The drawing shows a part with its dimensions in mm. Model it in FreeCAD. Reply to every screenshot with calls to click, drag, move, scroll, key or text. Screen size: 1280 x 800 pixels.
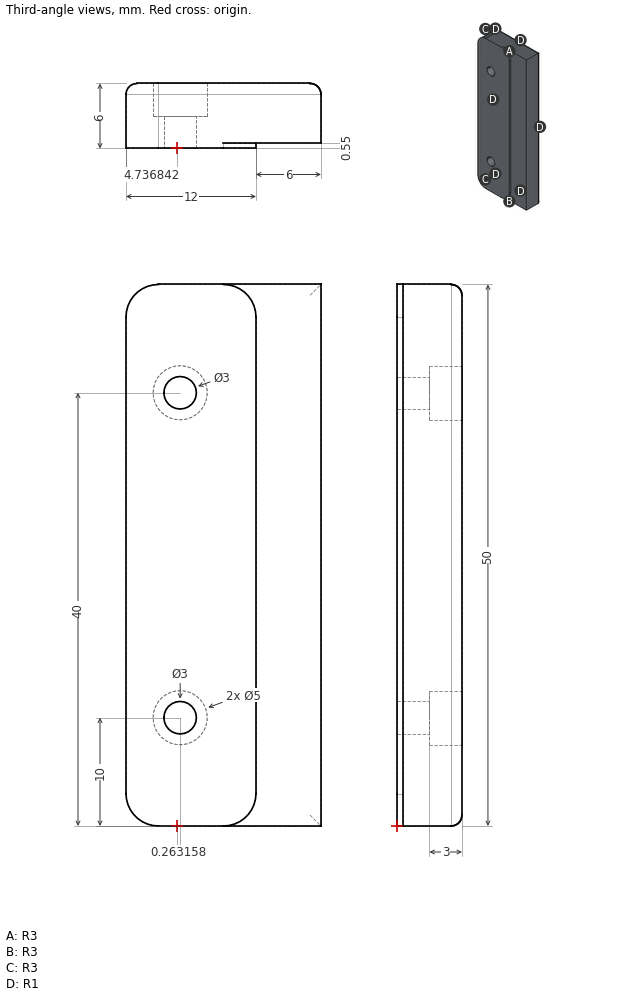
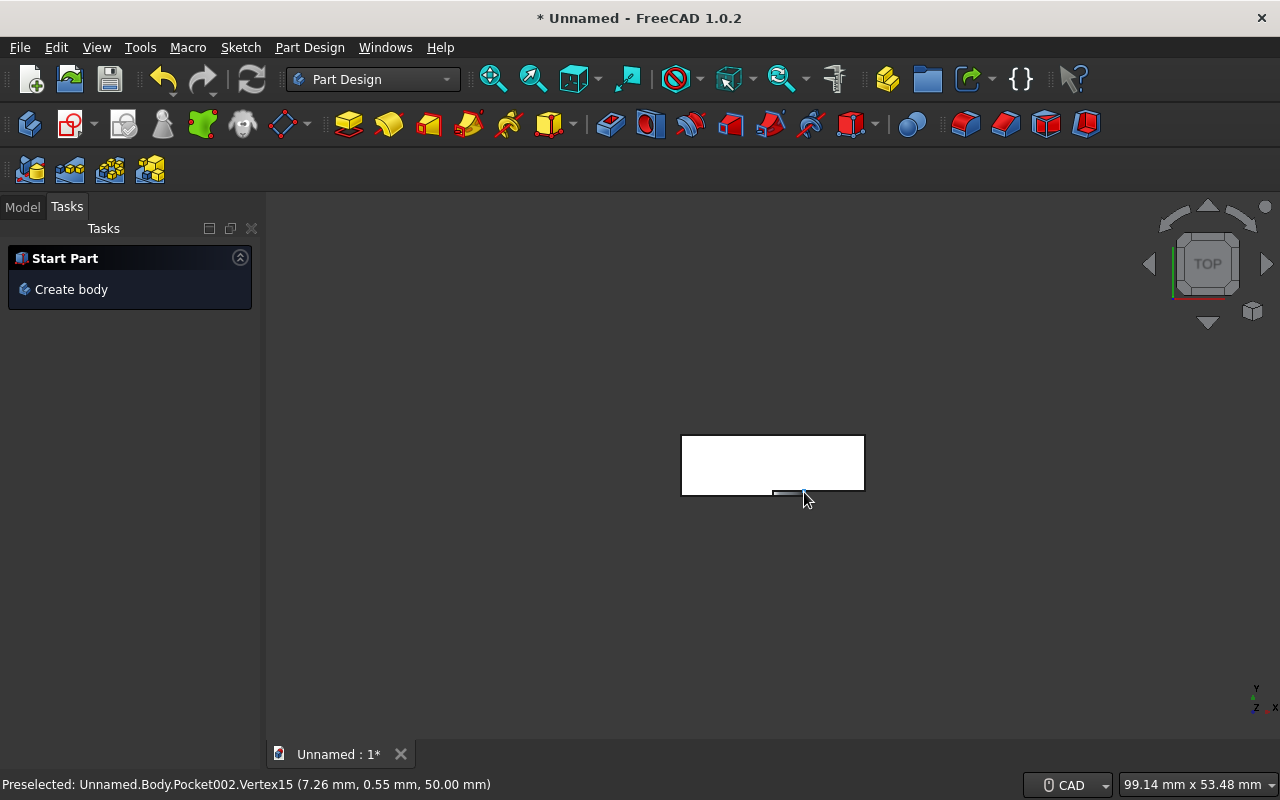
key(1)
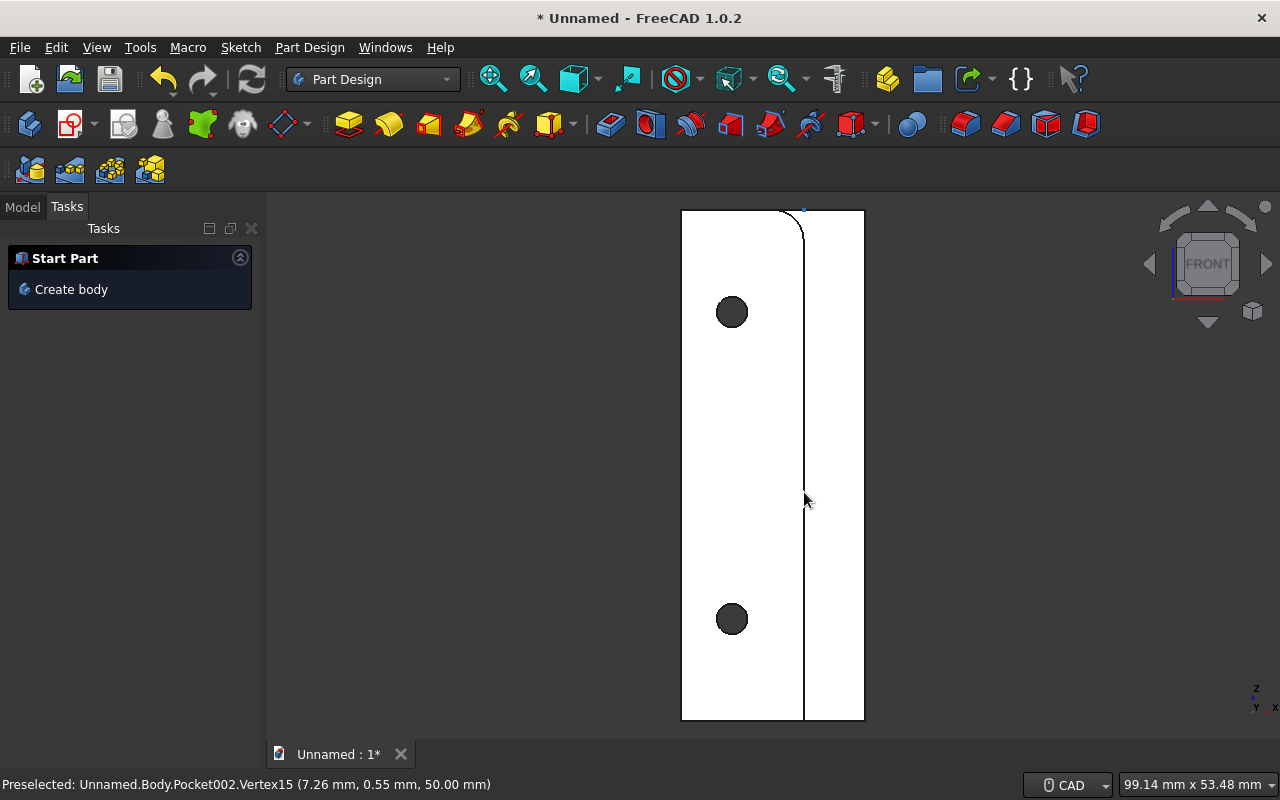
key(3)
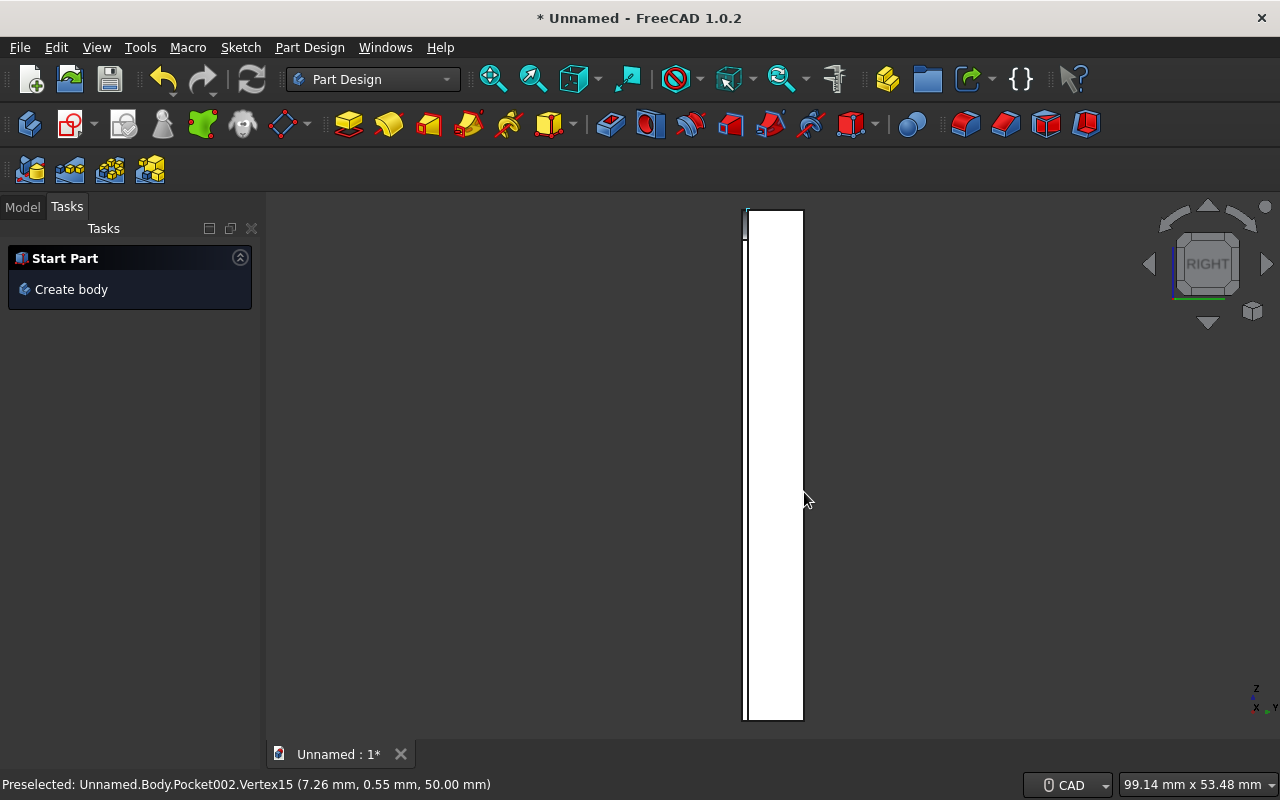
key(5)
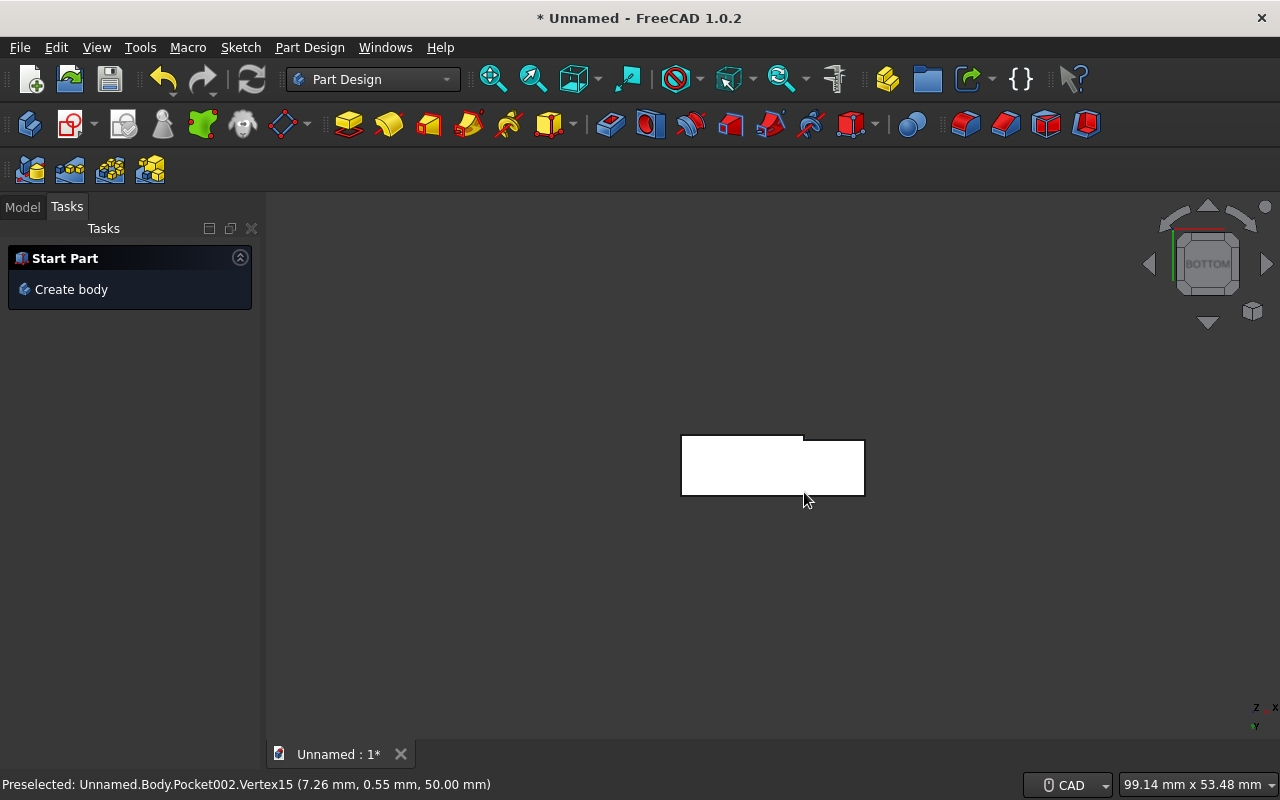
click(494, 80)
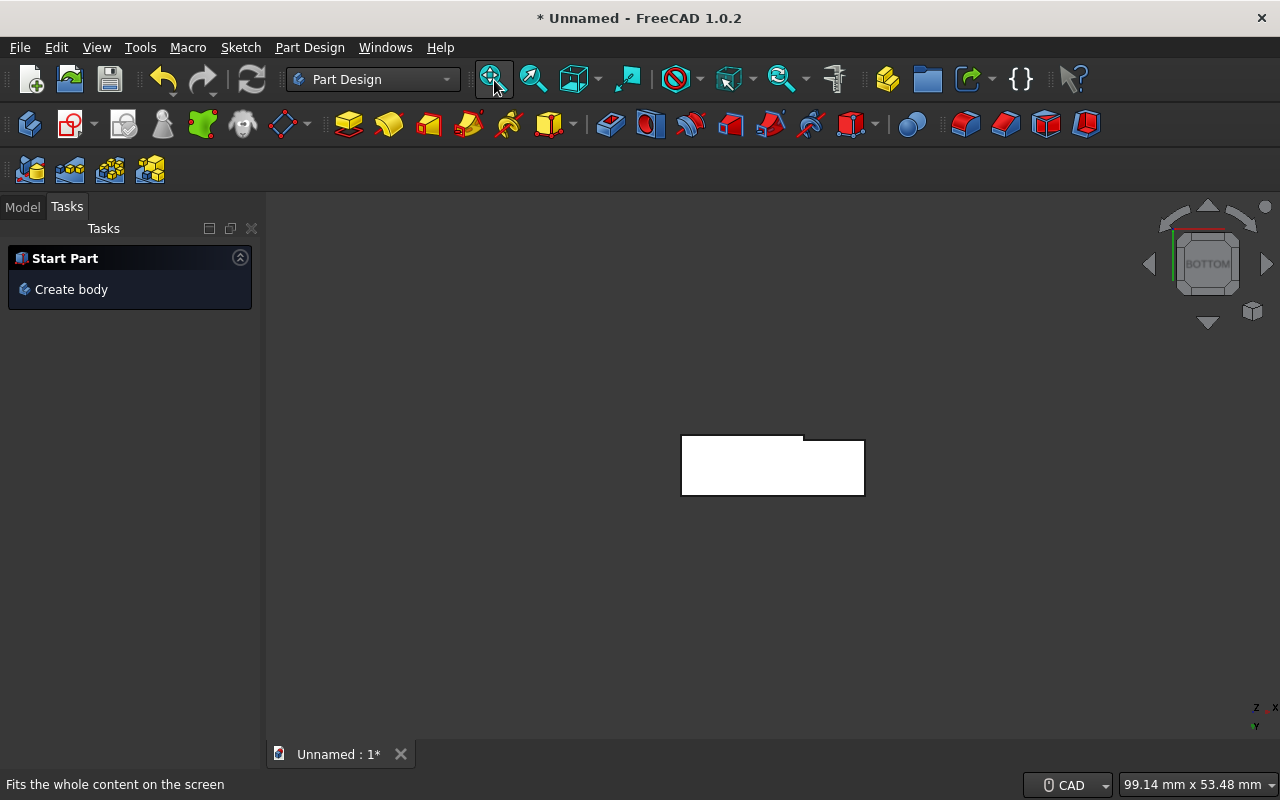
scroll(804, 437, up, 10)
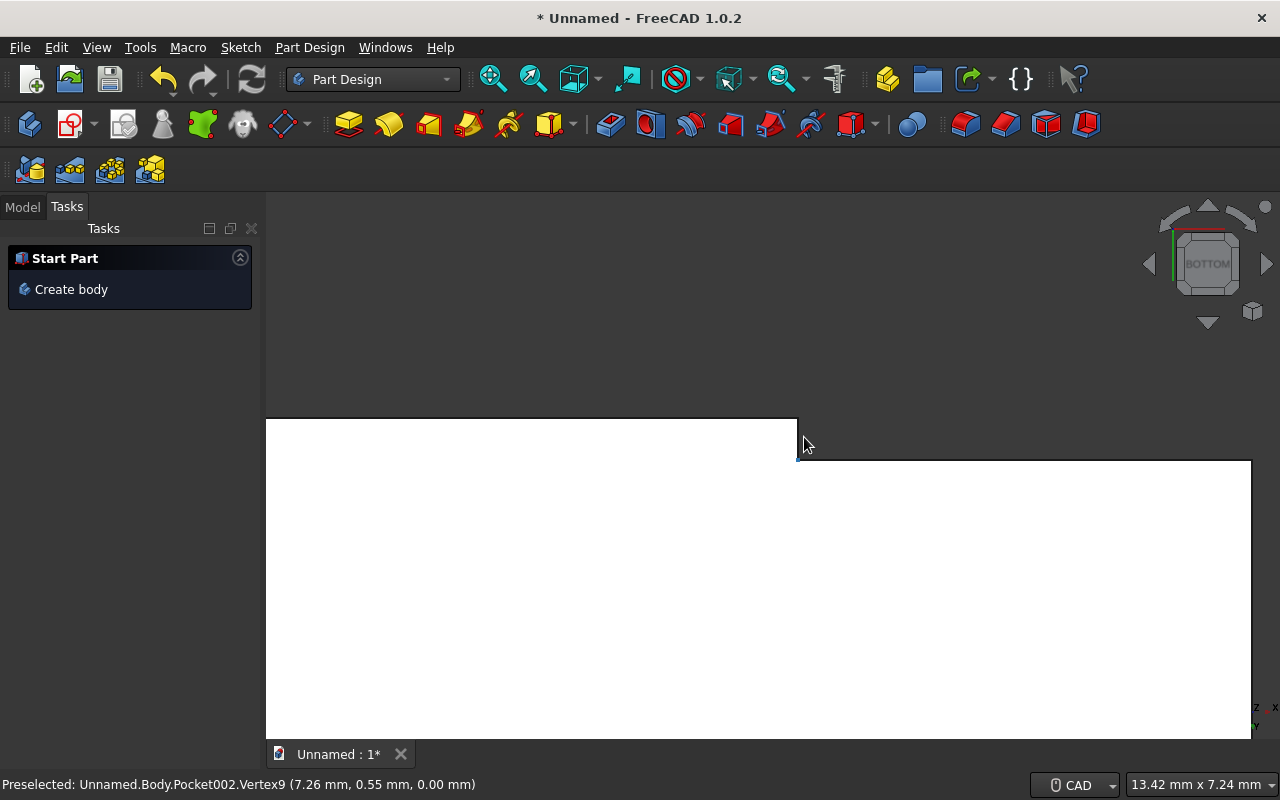
click(798, 438)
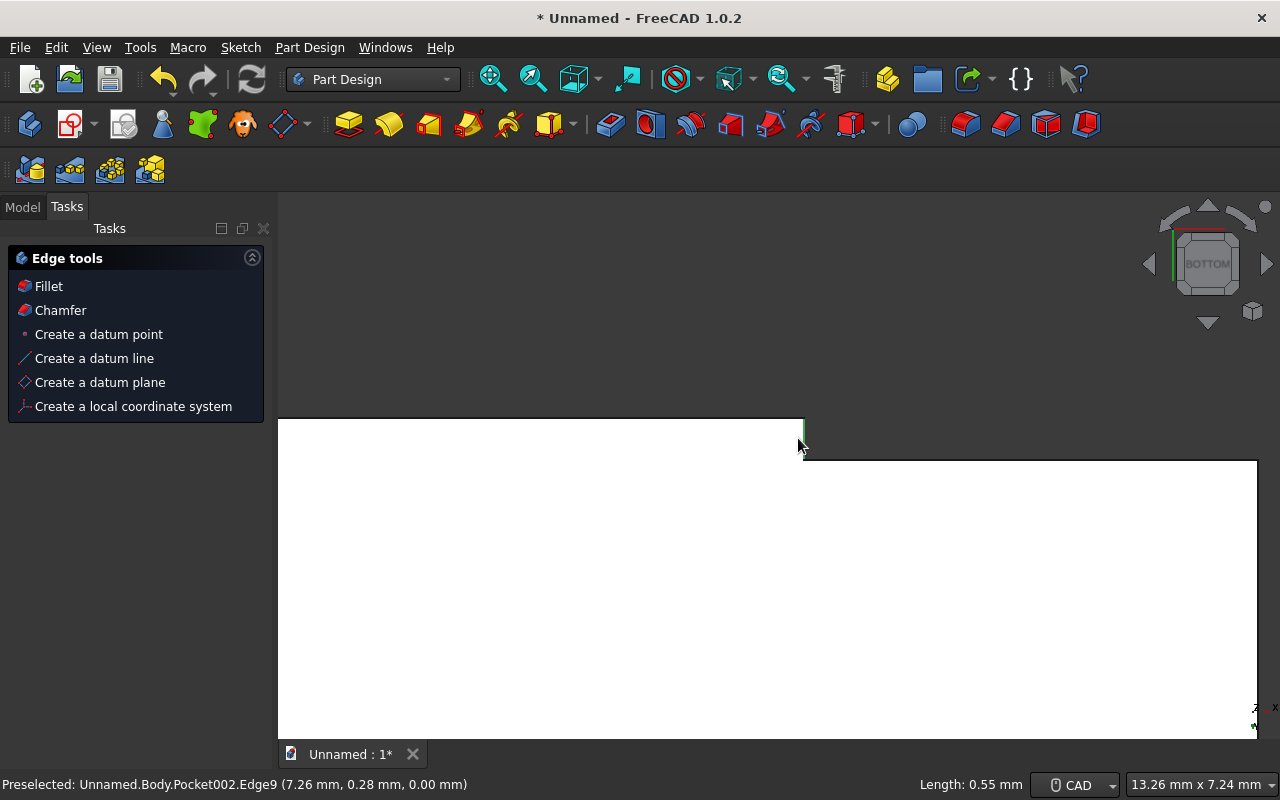
click(966, 124)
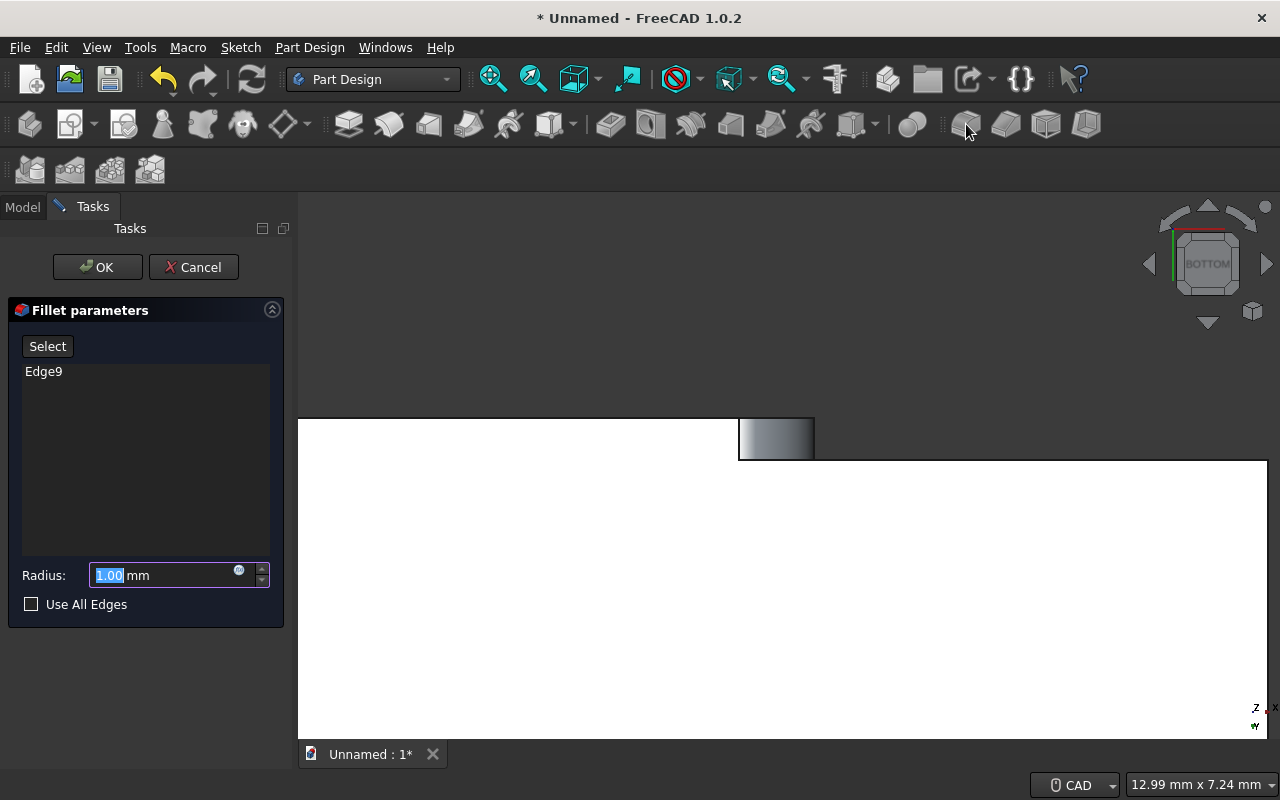
text(3)
key(Tab)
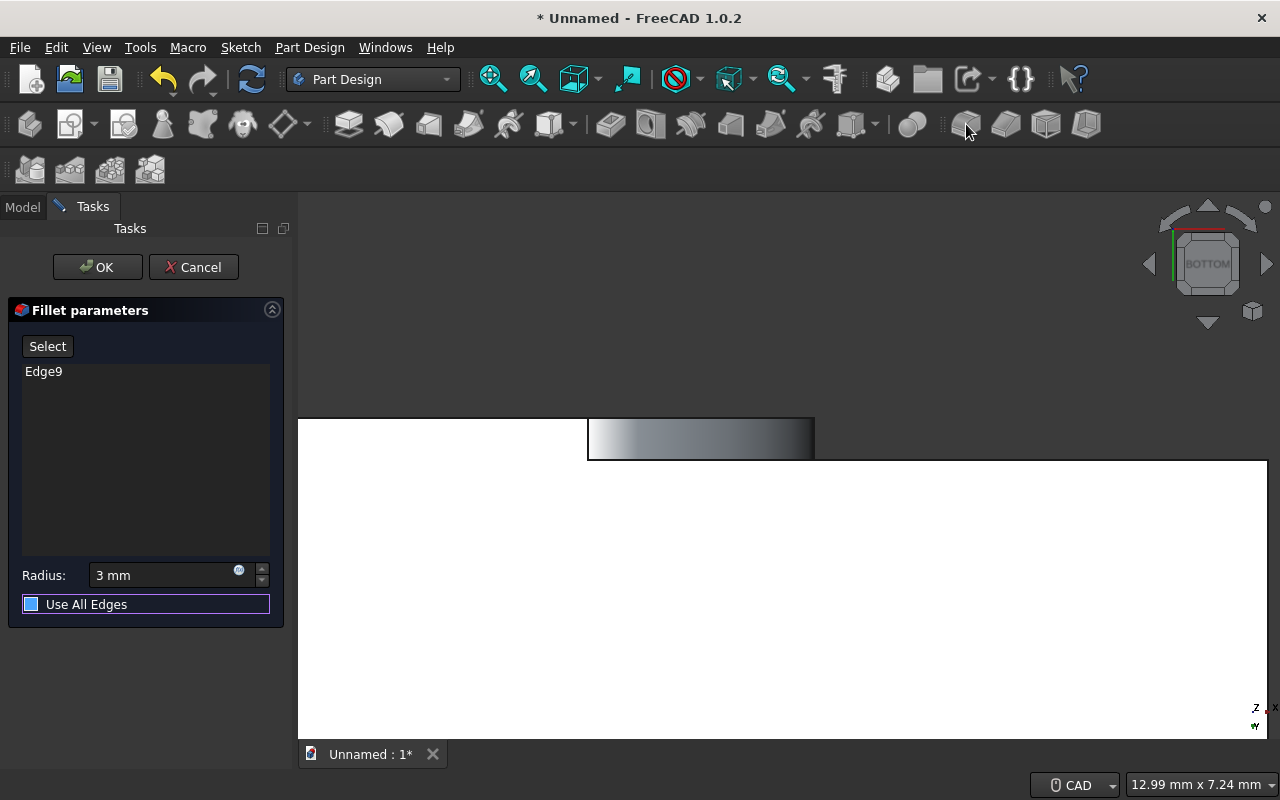
click(98, 267)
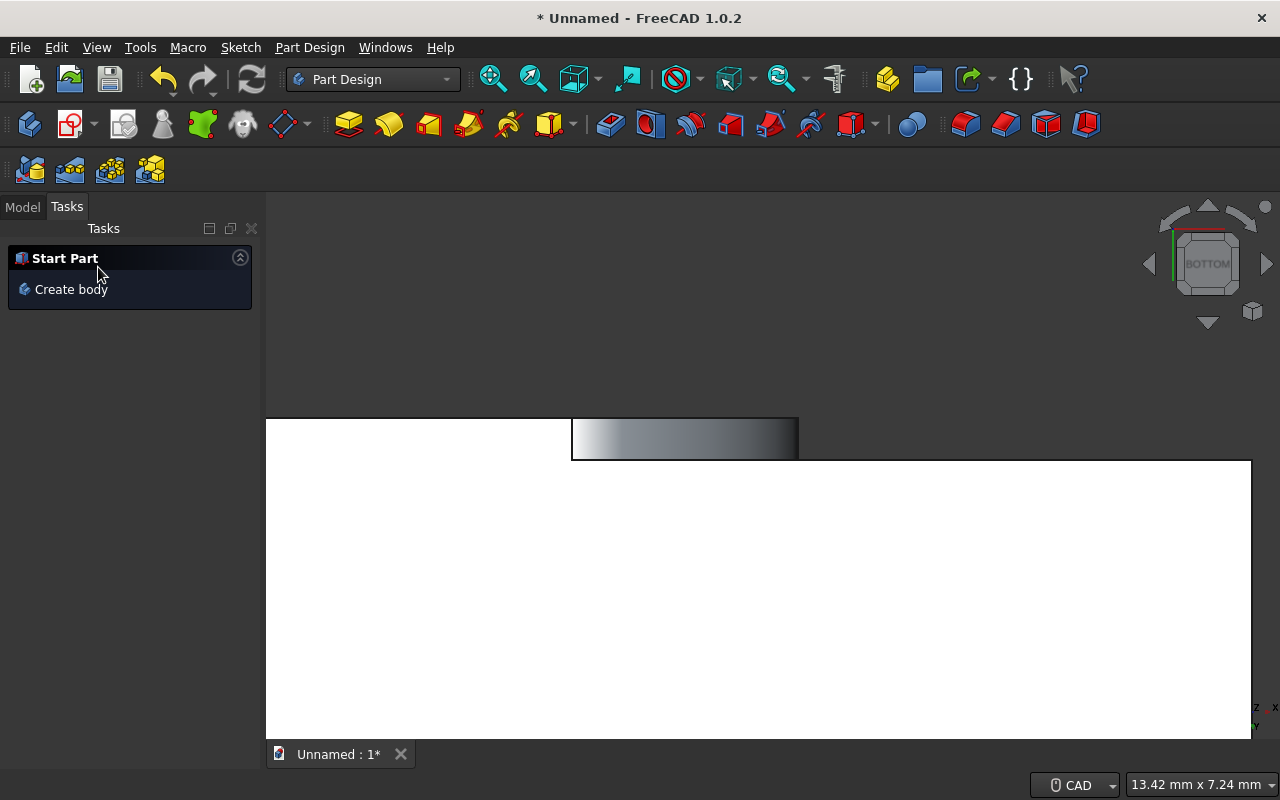
click(494, 80)